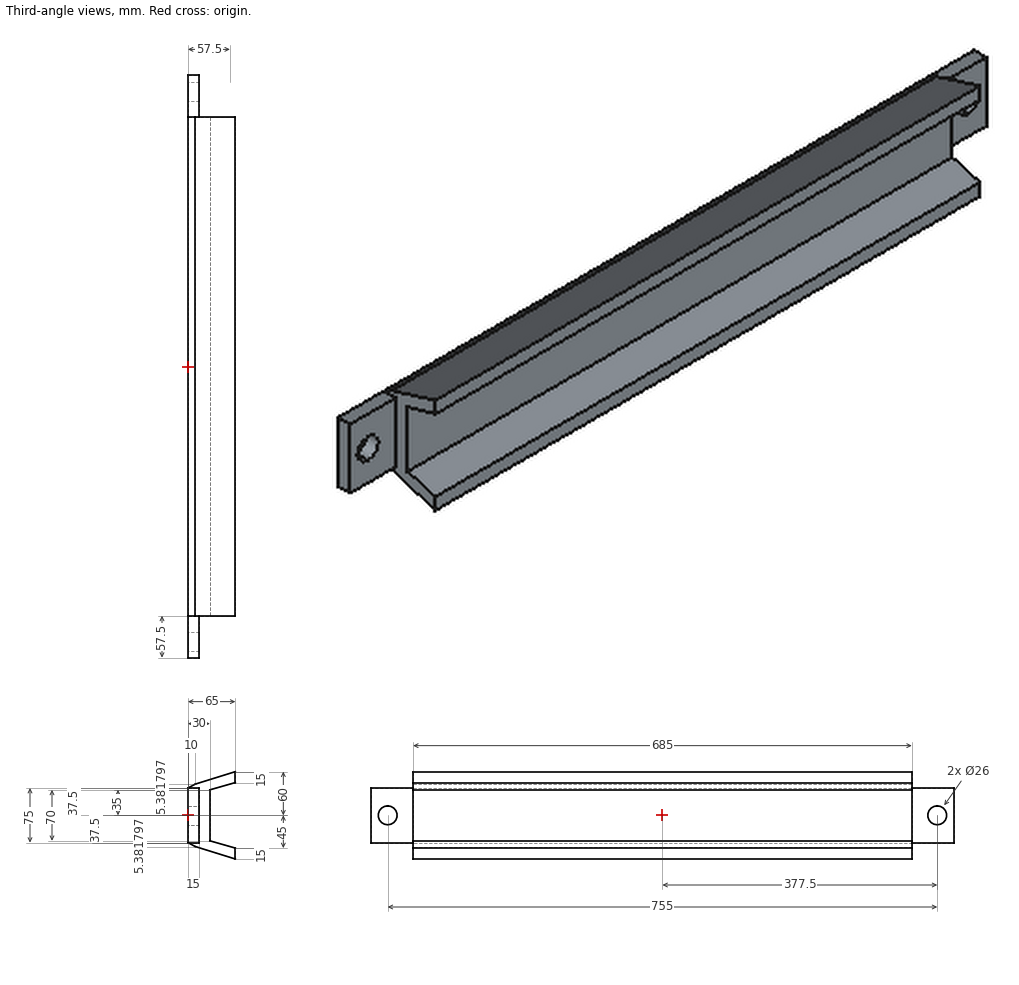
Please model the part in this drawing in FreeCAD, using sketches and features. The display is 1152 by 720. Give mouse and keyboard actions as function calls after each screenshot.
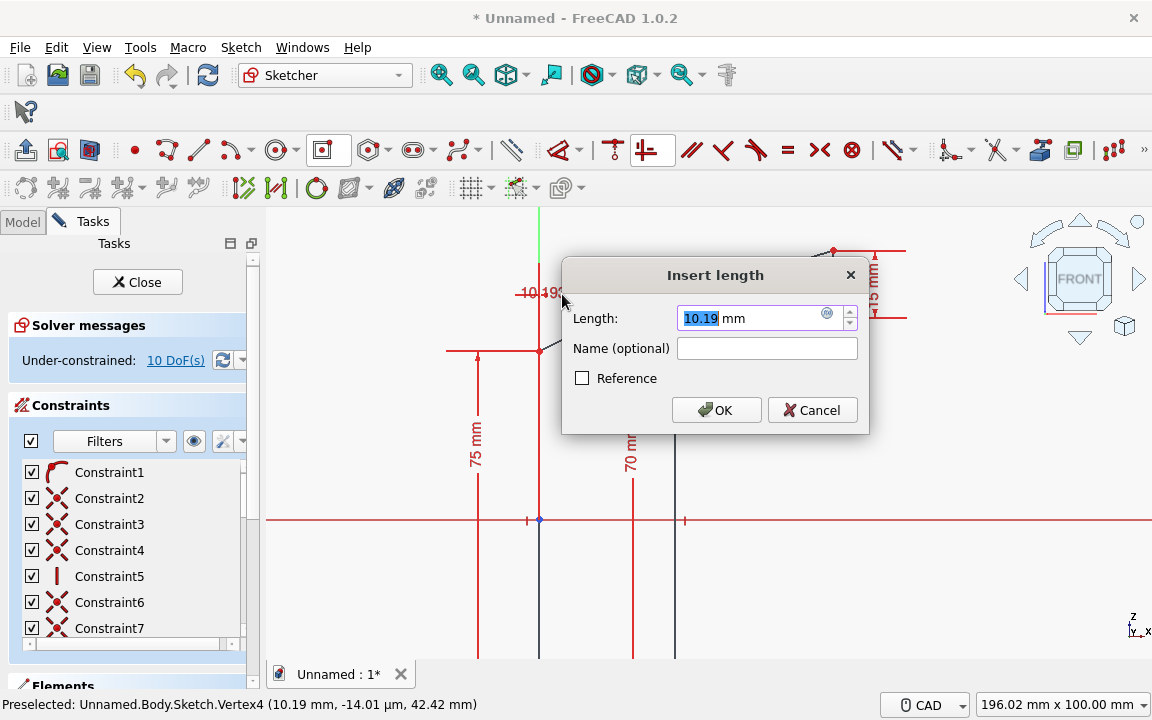
text(10)
key(Return)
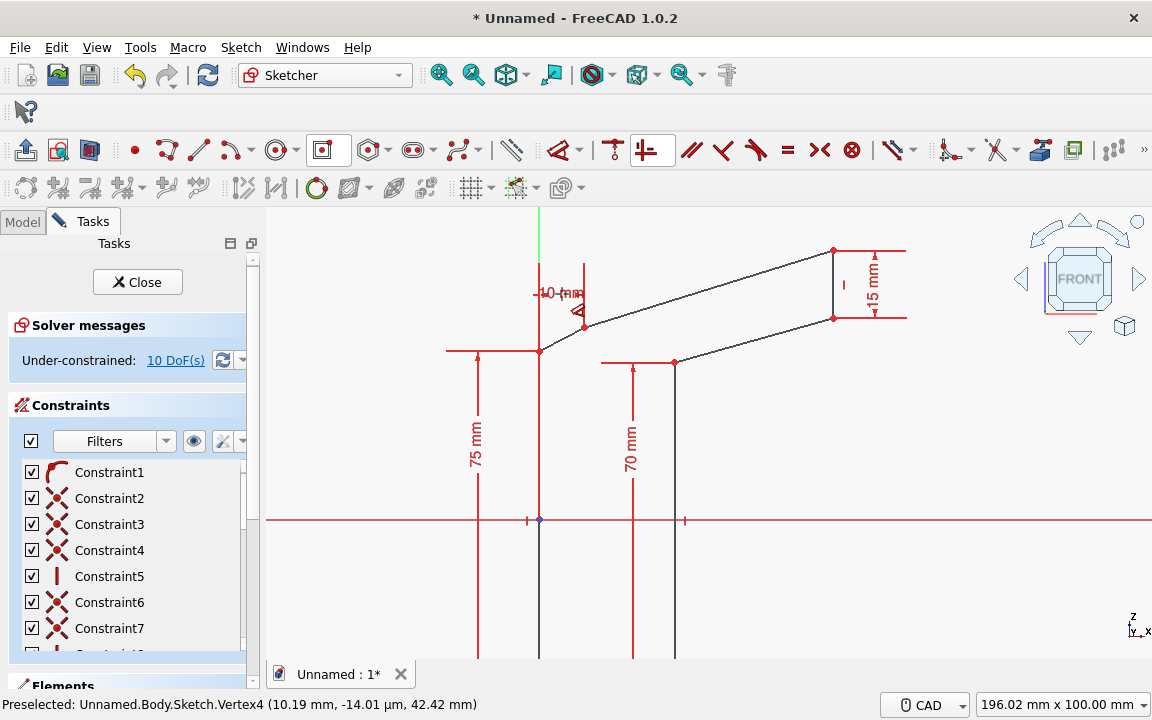
click(833, 251)
click(619, 554)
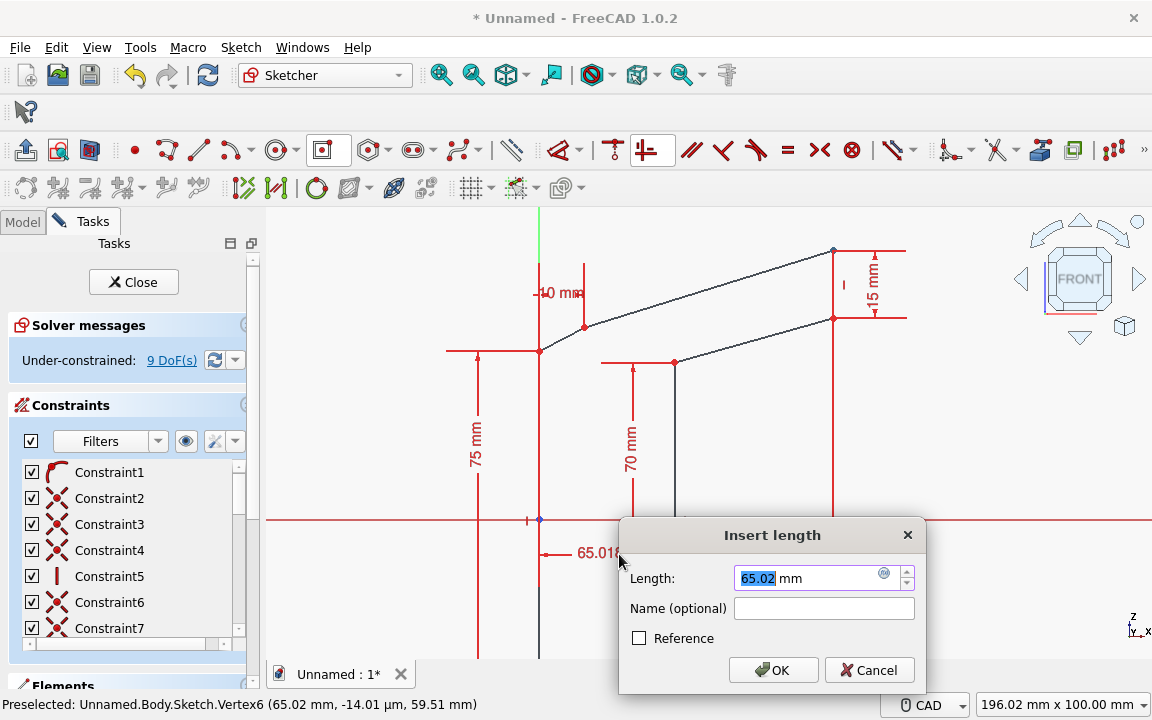
text(65)
key(Return)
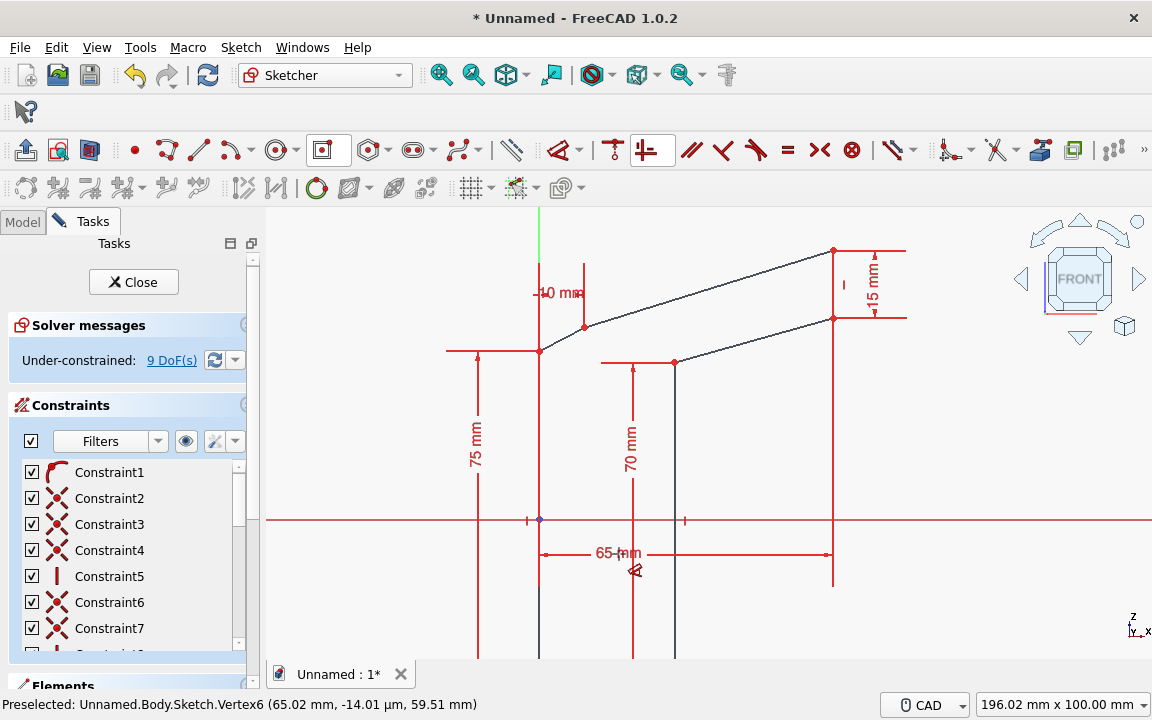
click(833, 251)
click(867, 385)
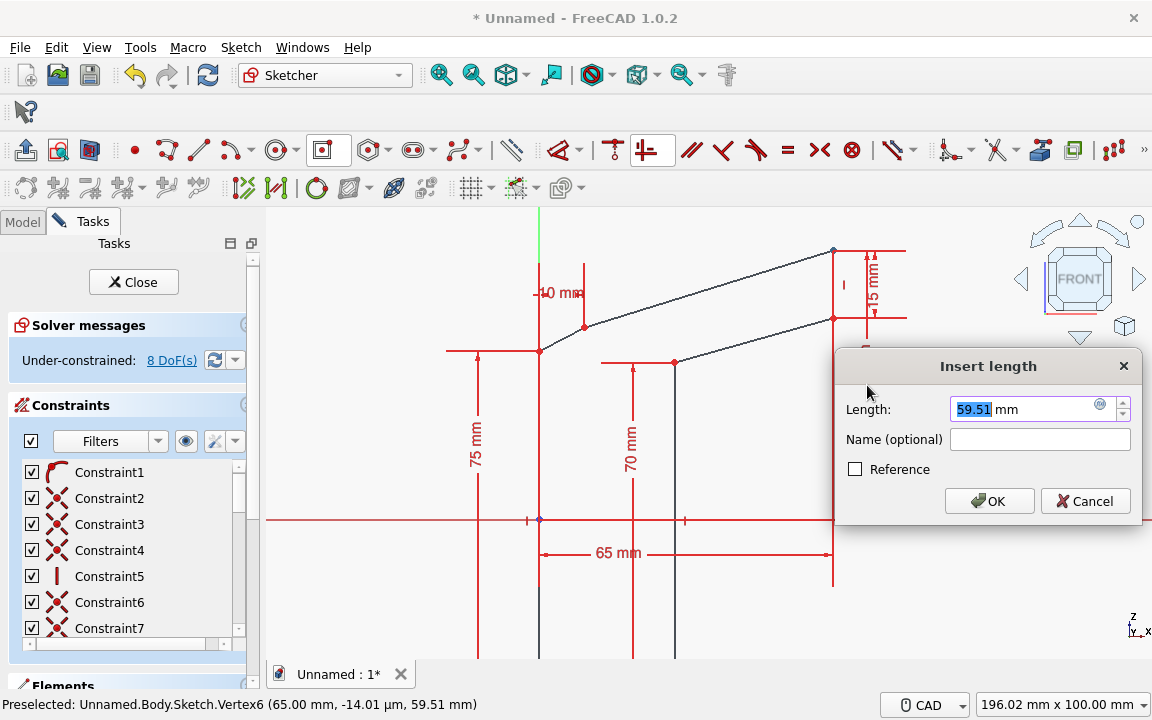
text(60)
key(Return)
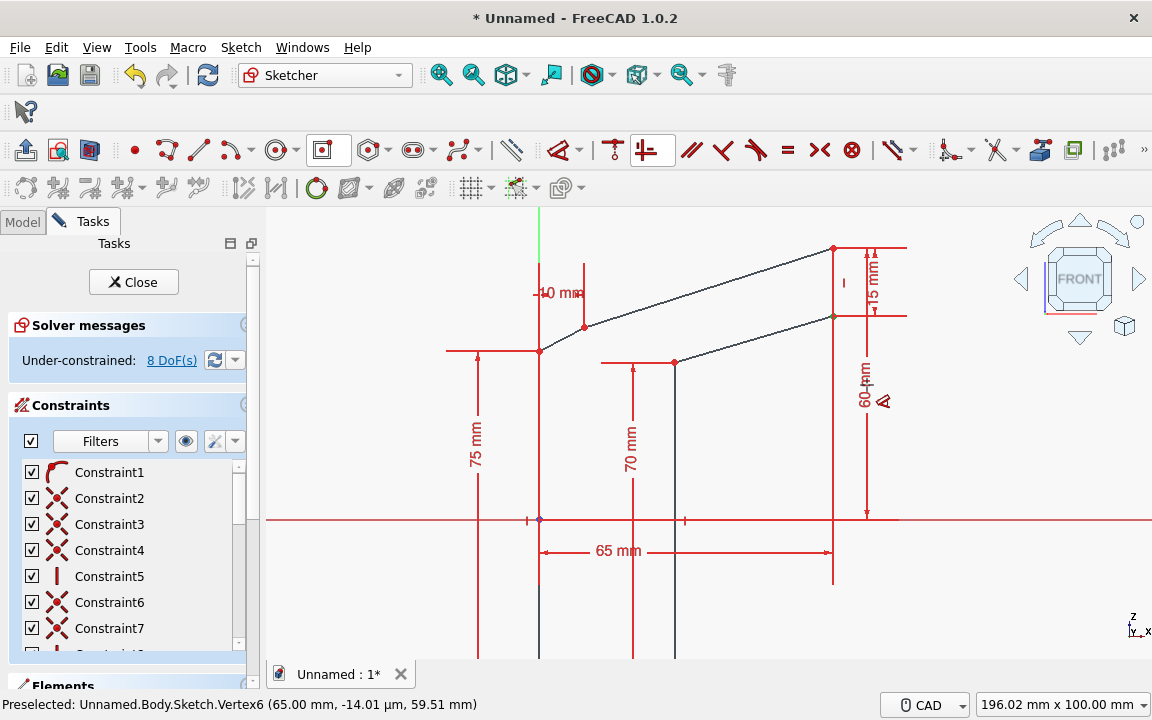
click(675, 363)
click(638, 329)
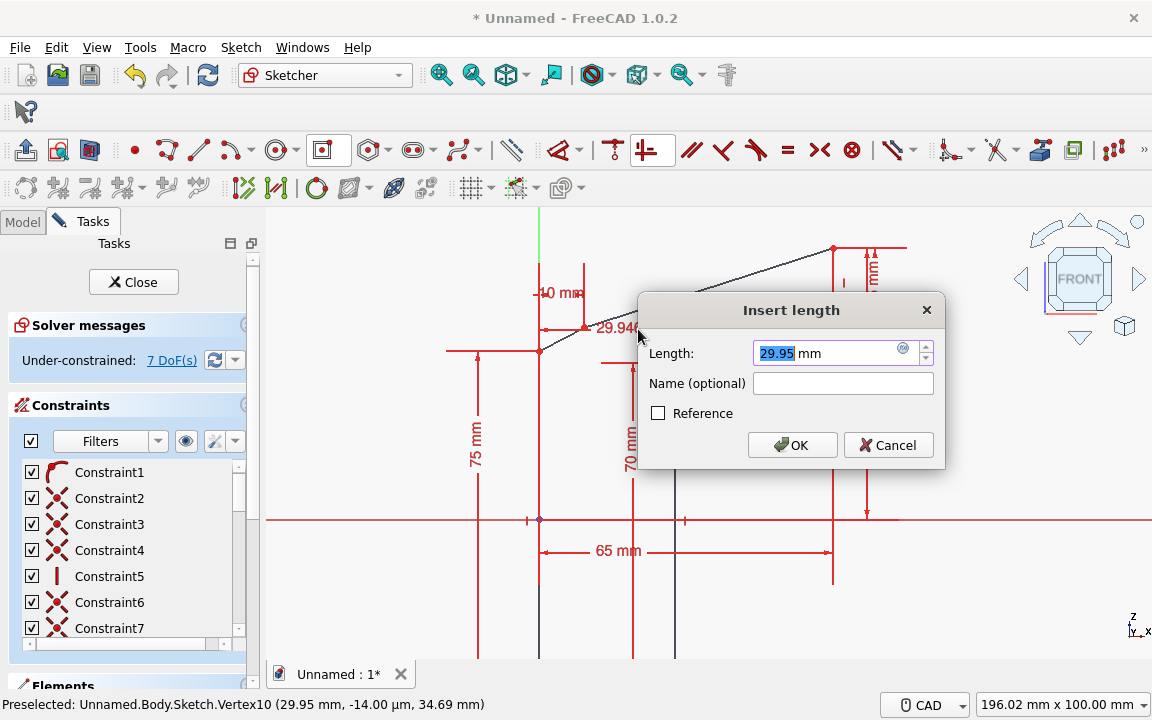
text(30)
key(Return)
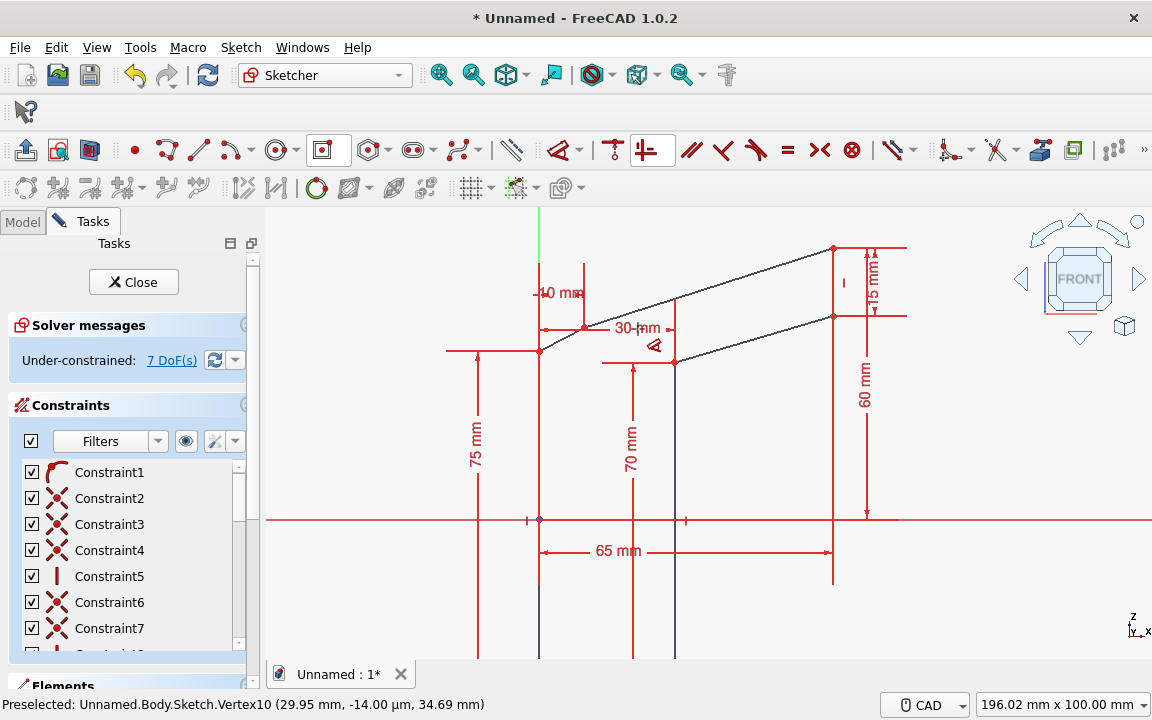
click(675, 363)
click(505, 405)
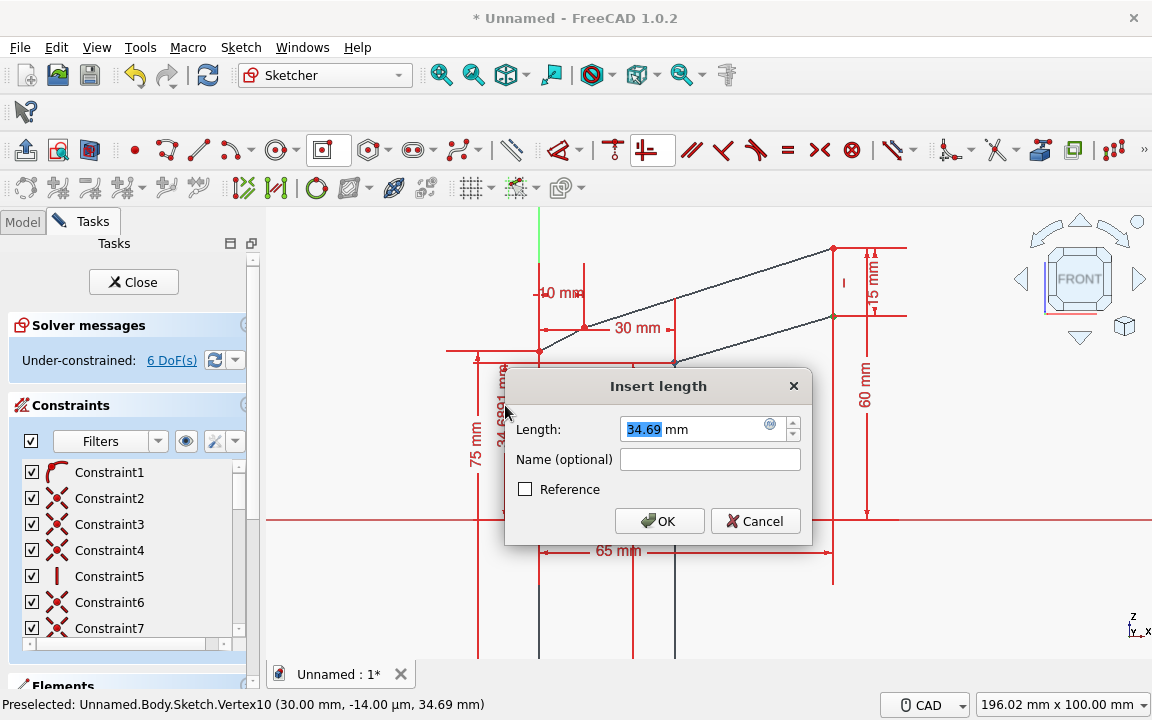
text(35)
key(Return)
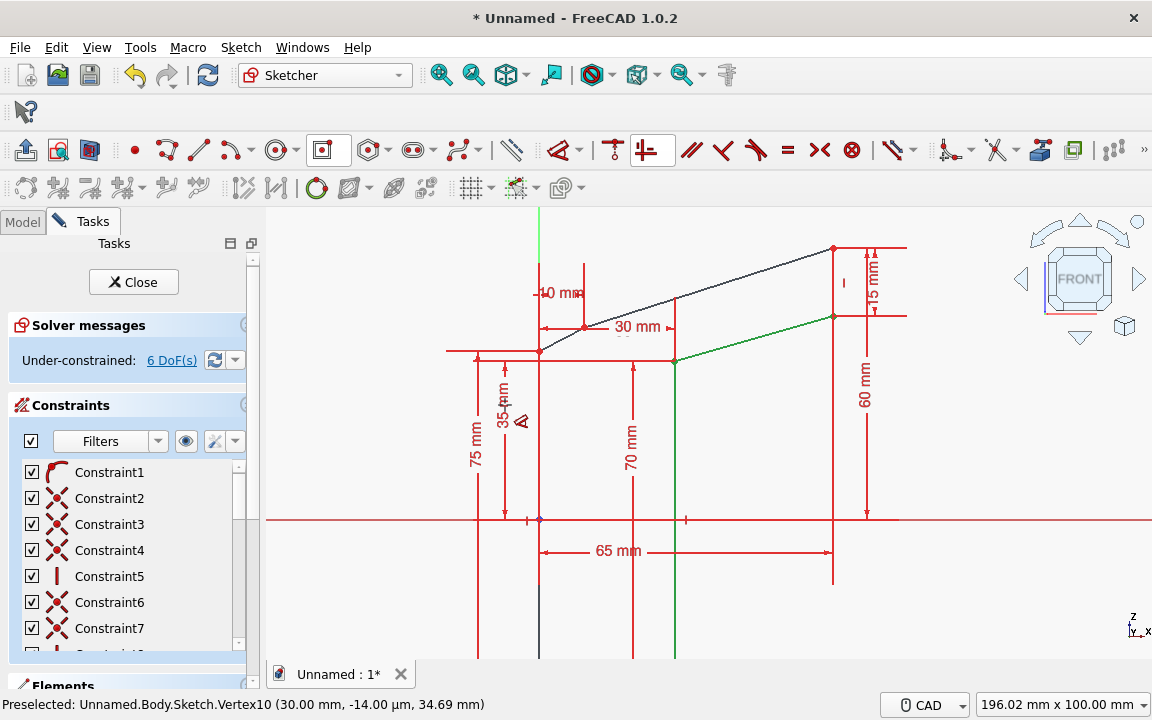
scroll(585, 328, down, 3)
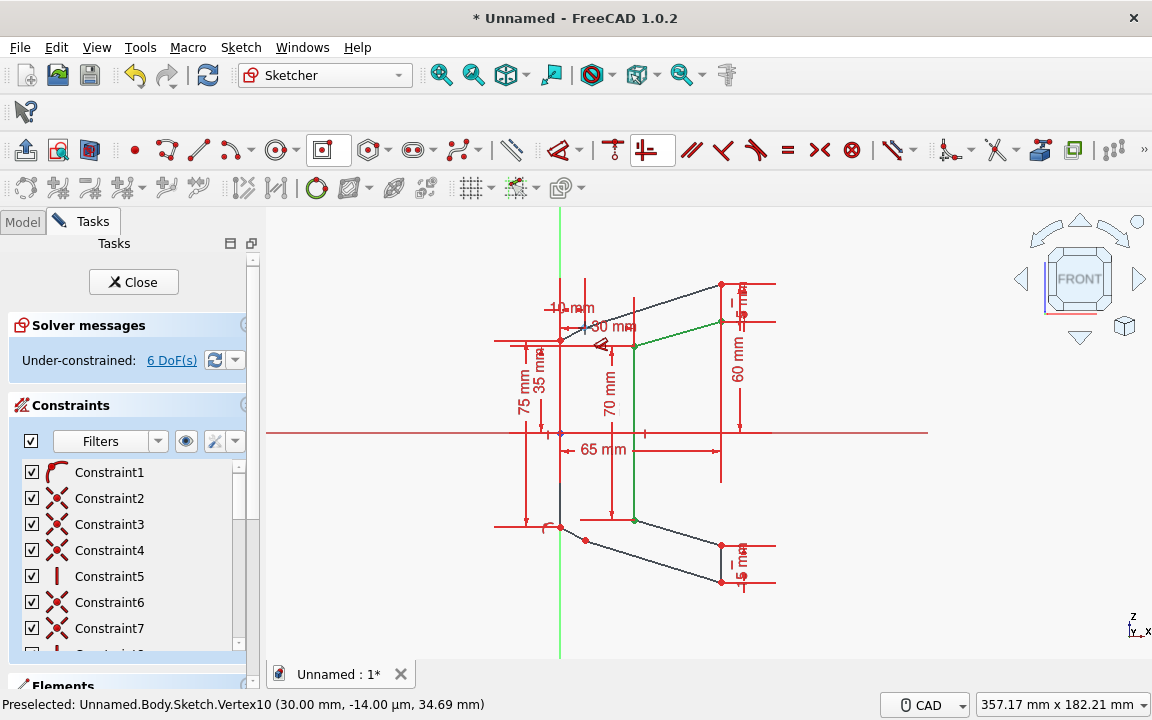
click(721, 546)
click(641, 580)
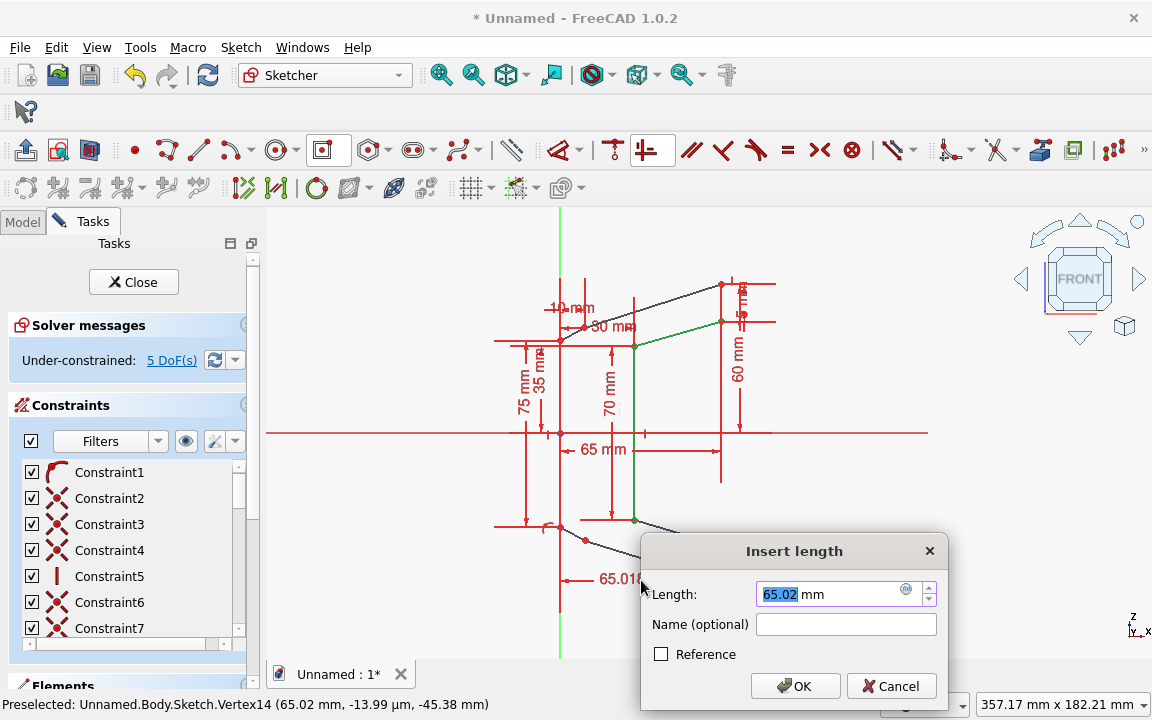
text(65)
key(Return)